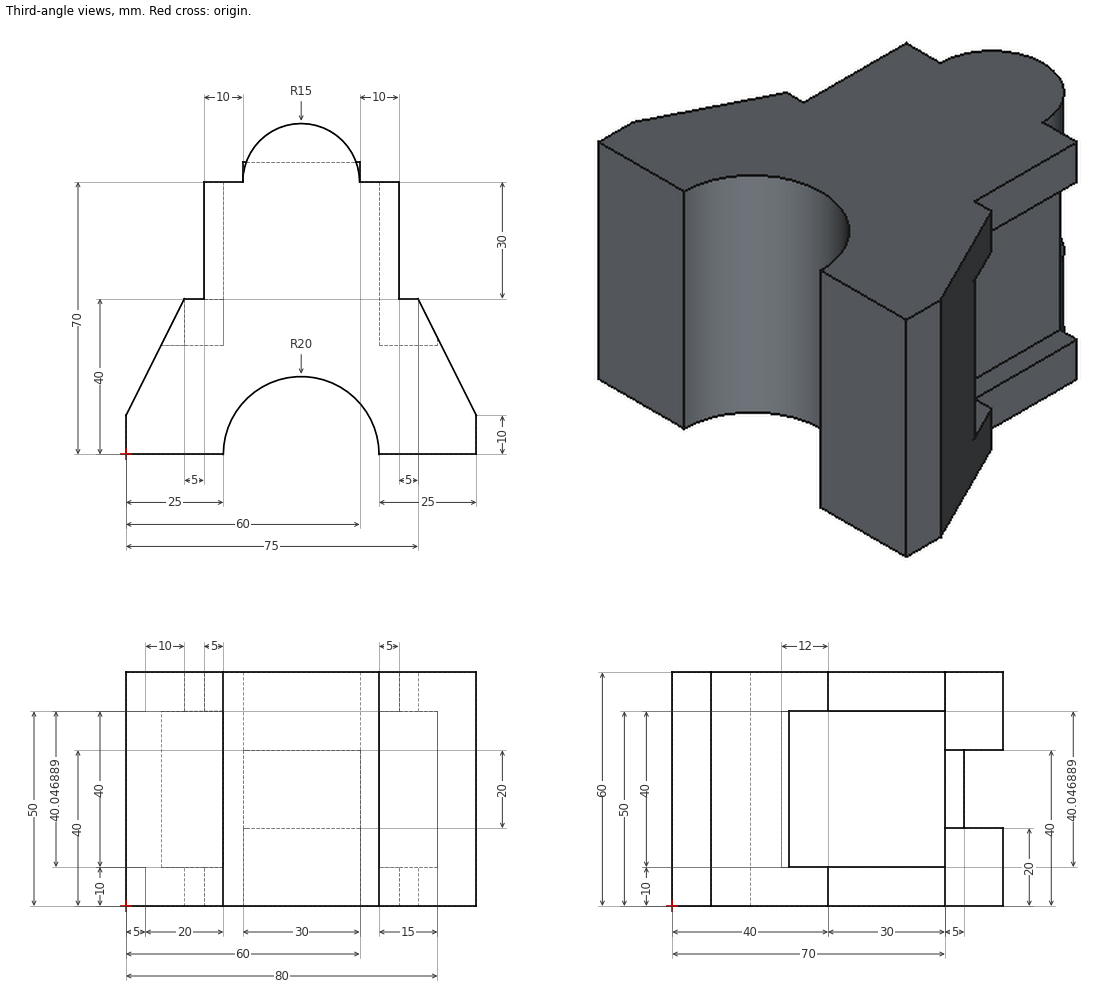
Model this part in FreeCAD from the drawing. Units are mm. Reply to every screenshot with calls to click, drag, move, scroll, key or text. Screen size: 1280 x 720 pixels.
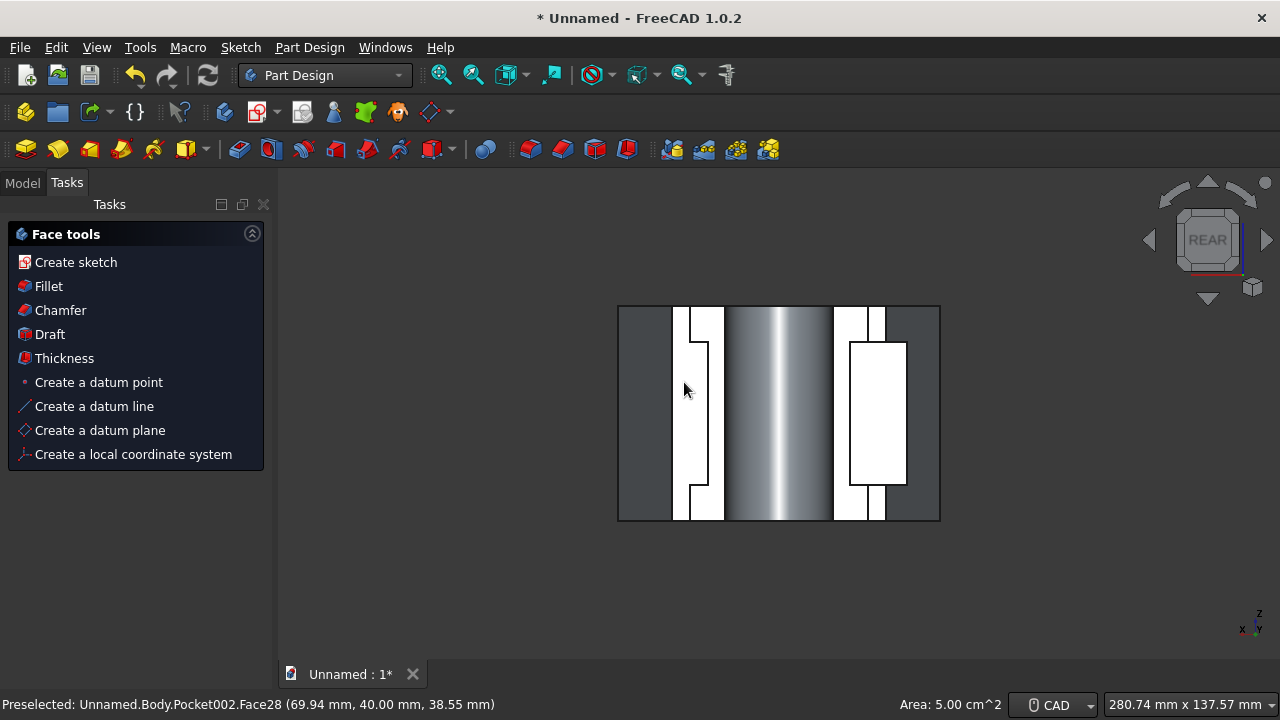
click(258, 112)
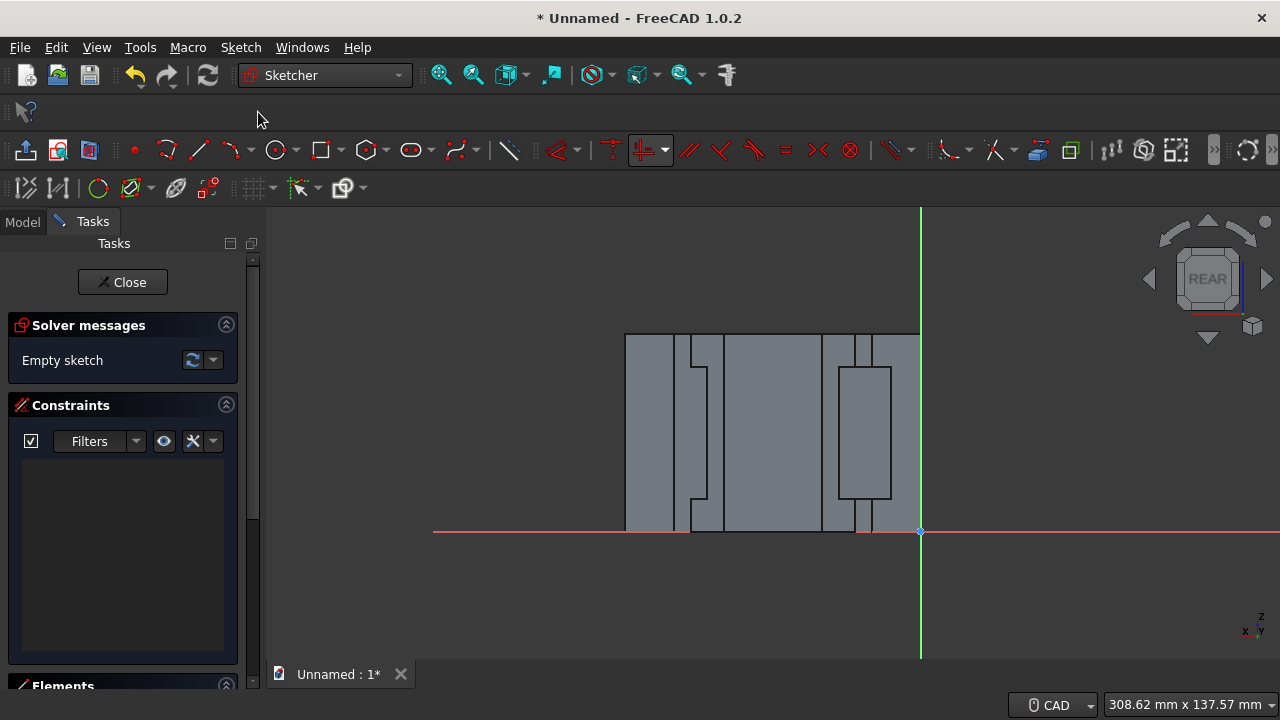
scroll(893, 469, up, 3)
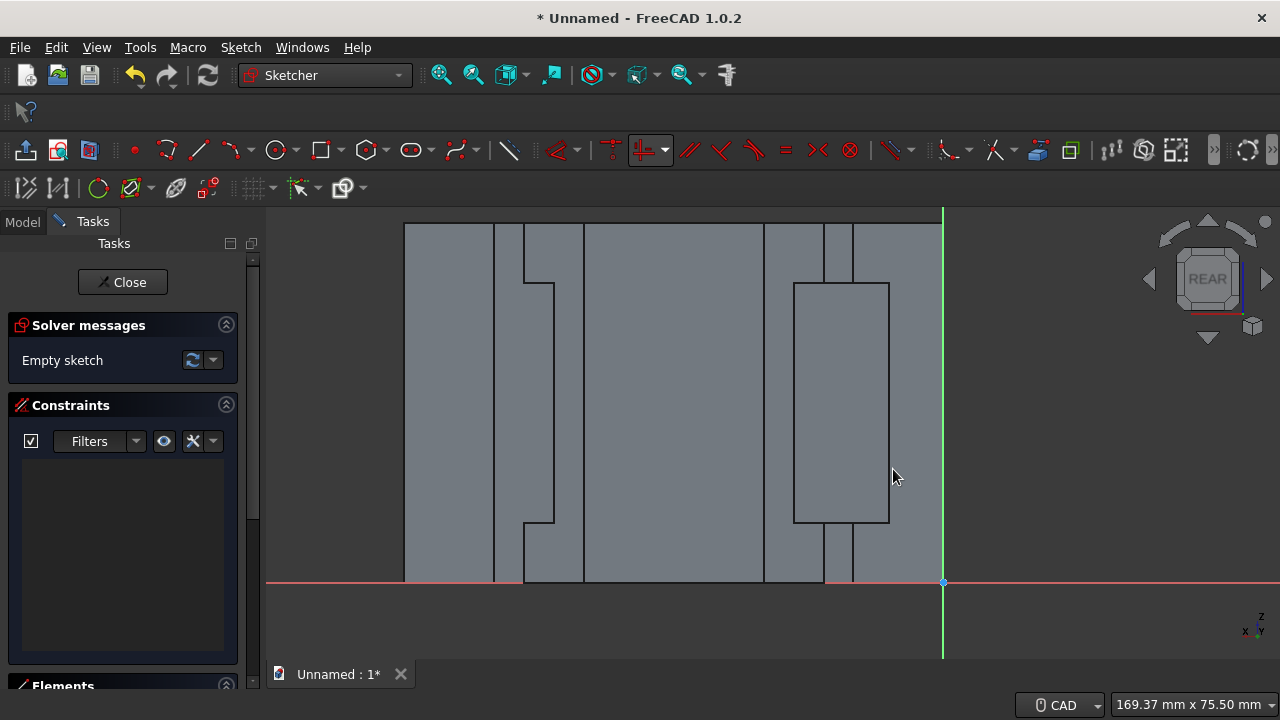
key(g)
key(r)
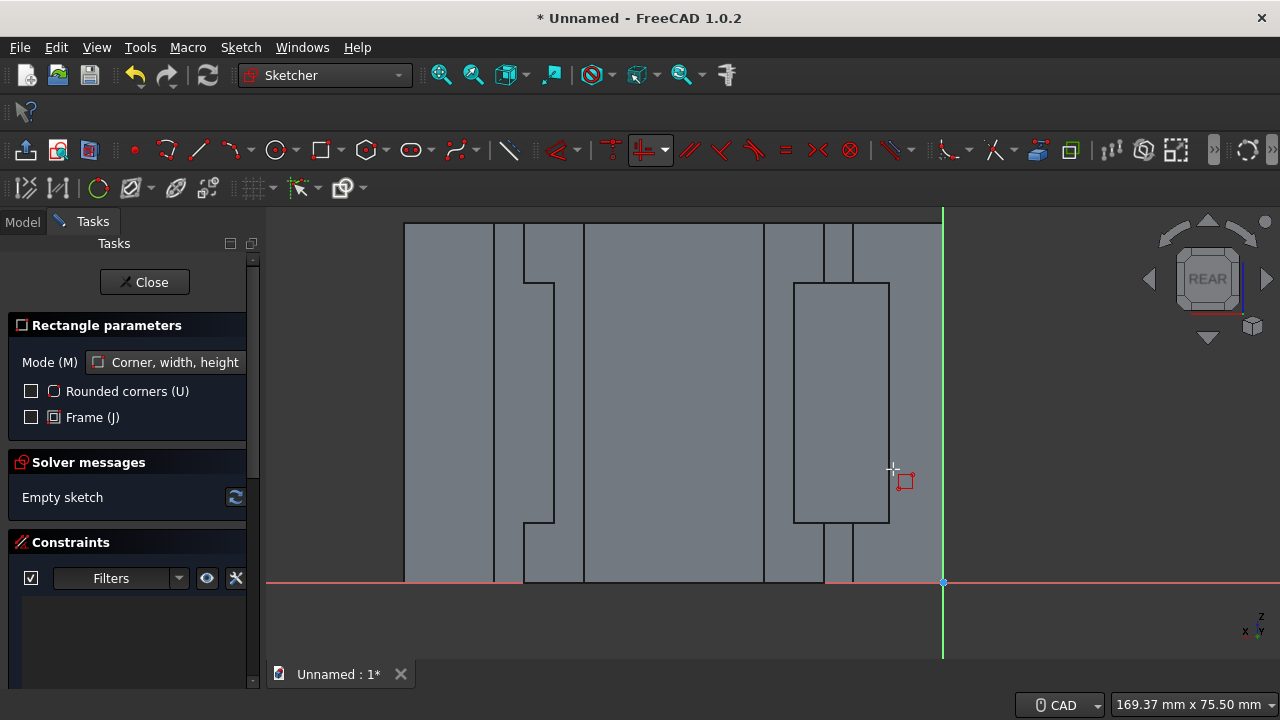
click(464, 283)
click(554, 523)
key(Escape)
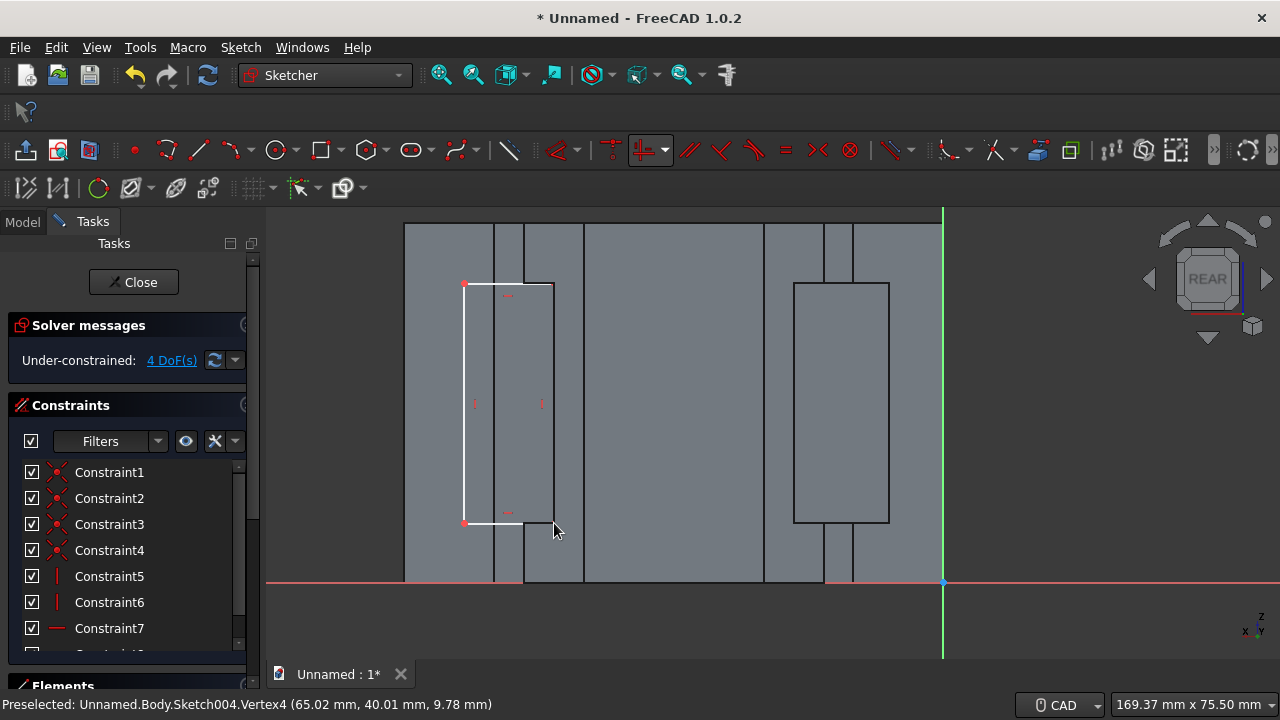
click(556, 150)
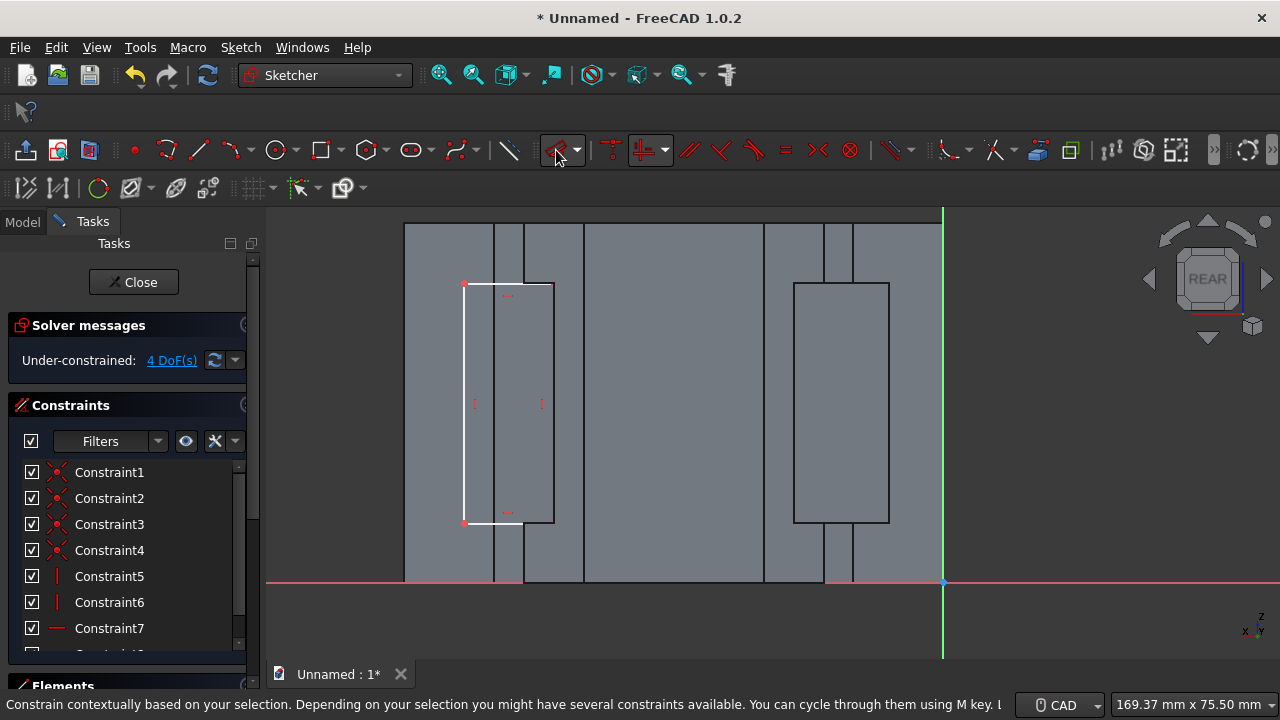
click(464, 356)
click(430, 404)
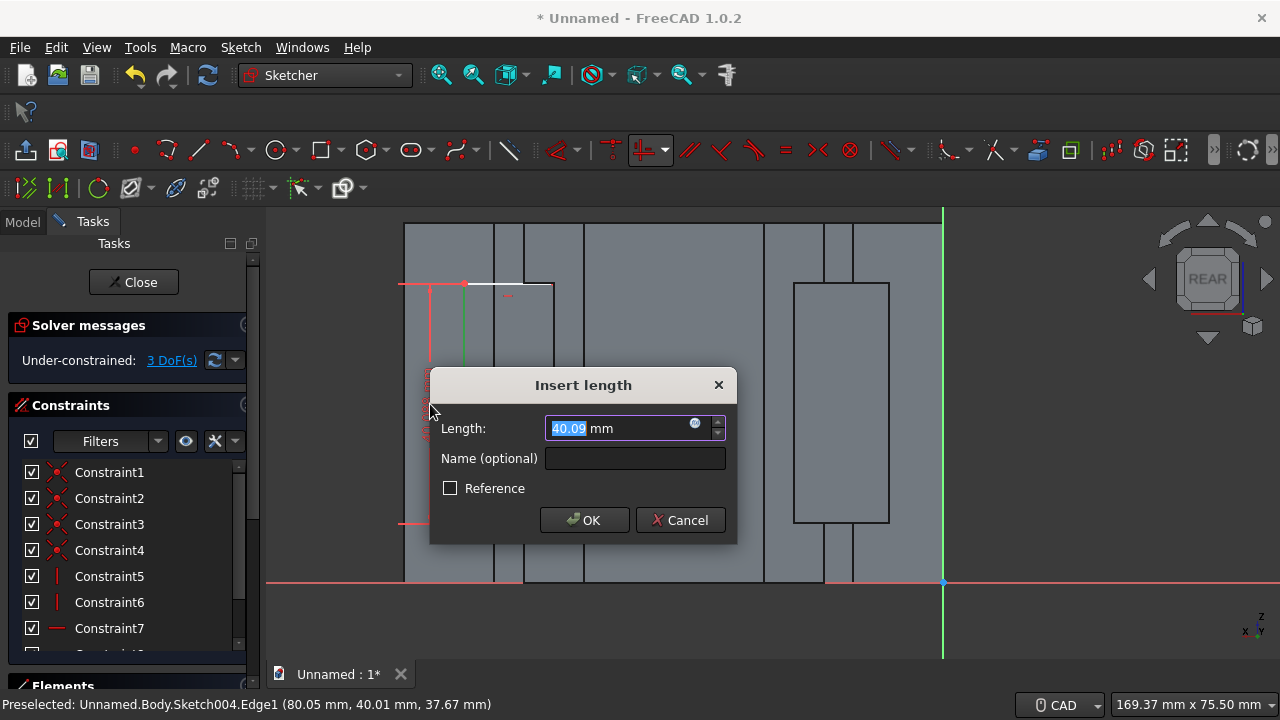
text(40)
key(Return)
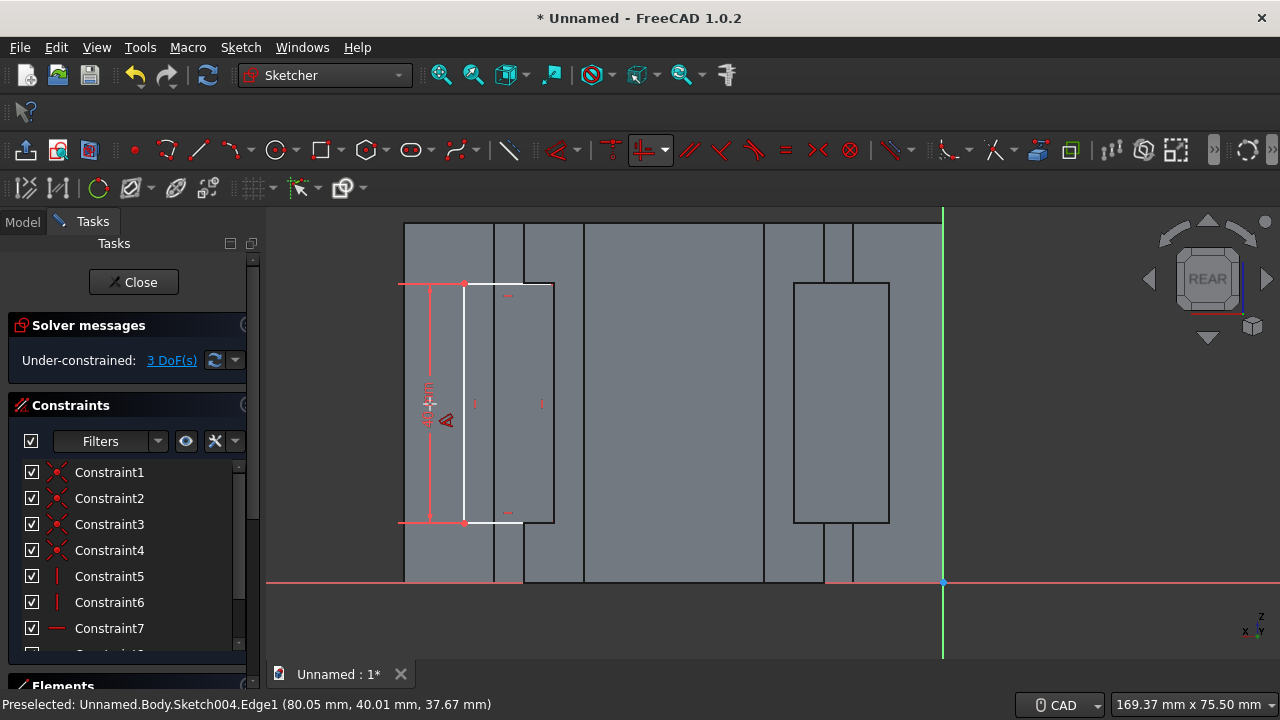
click(491, 523)
click(509, 557)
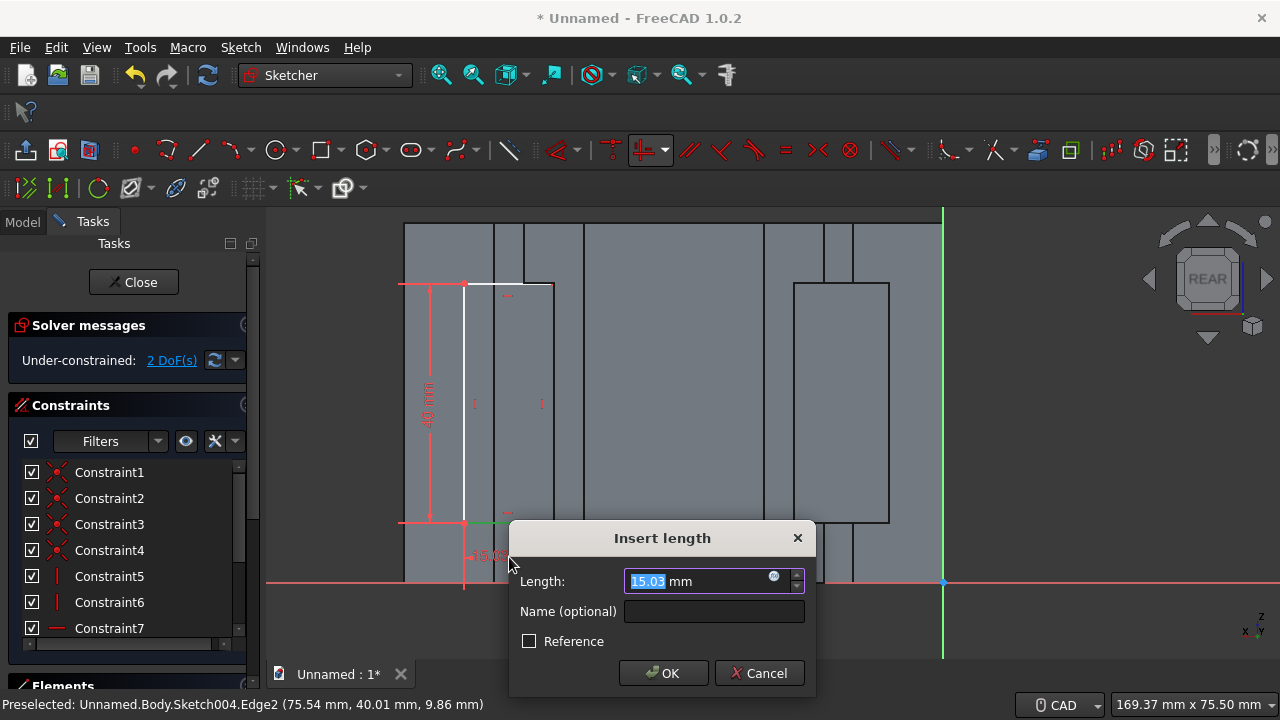
text(15)
key(Return)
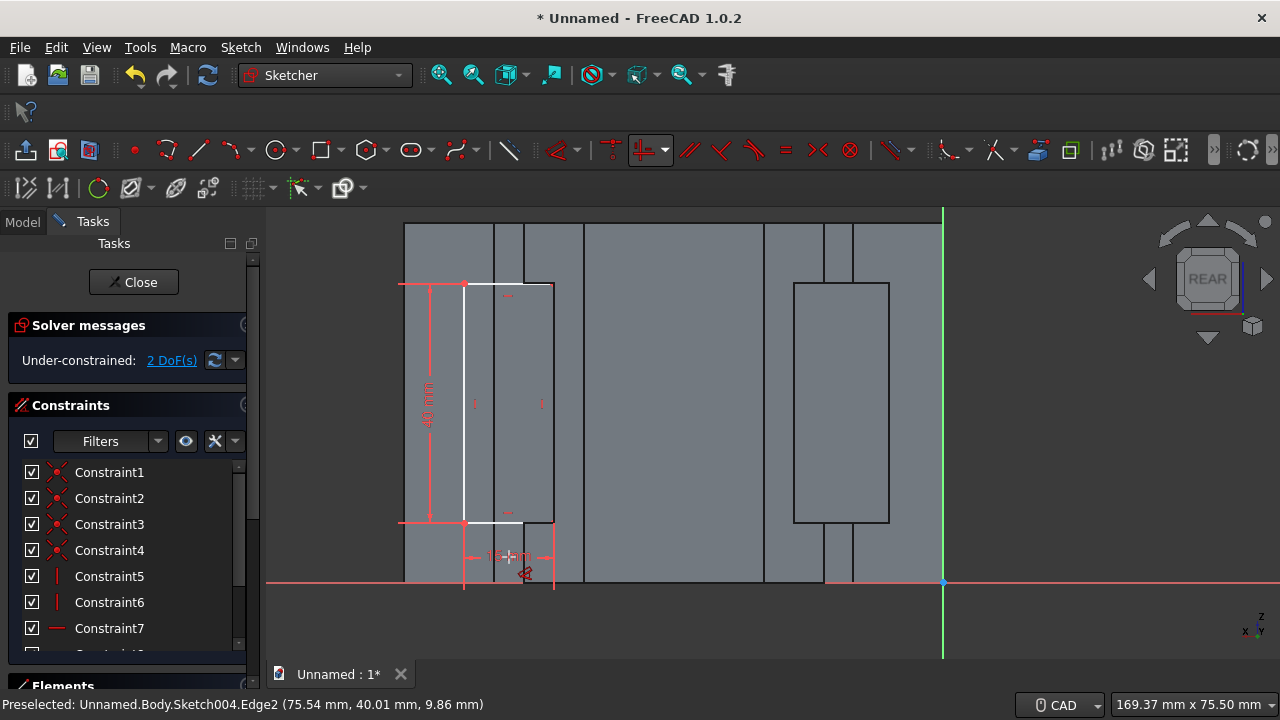
click(464, 284)
click(704, 617)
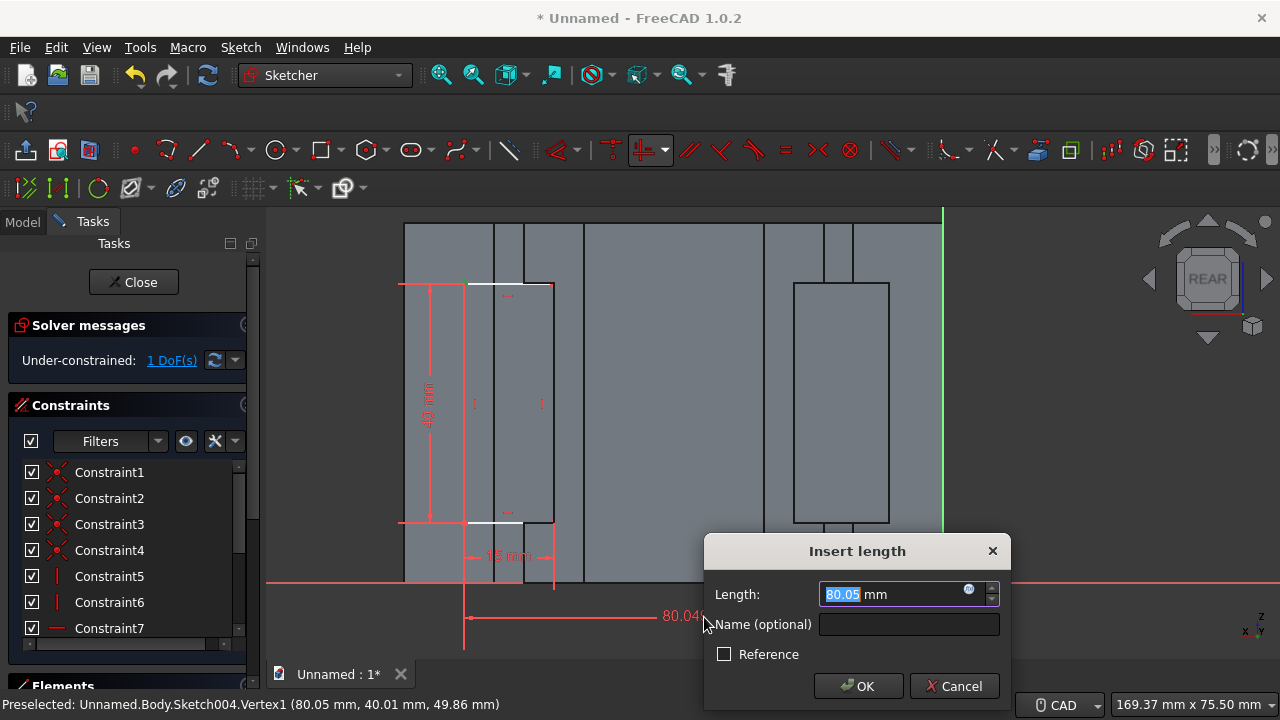
text(80)
key(Return)